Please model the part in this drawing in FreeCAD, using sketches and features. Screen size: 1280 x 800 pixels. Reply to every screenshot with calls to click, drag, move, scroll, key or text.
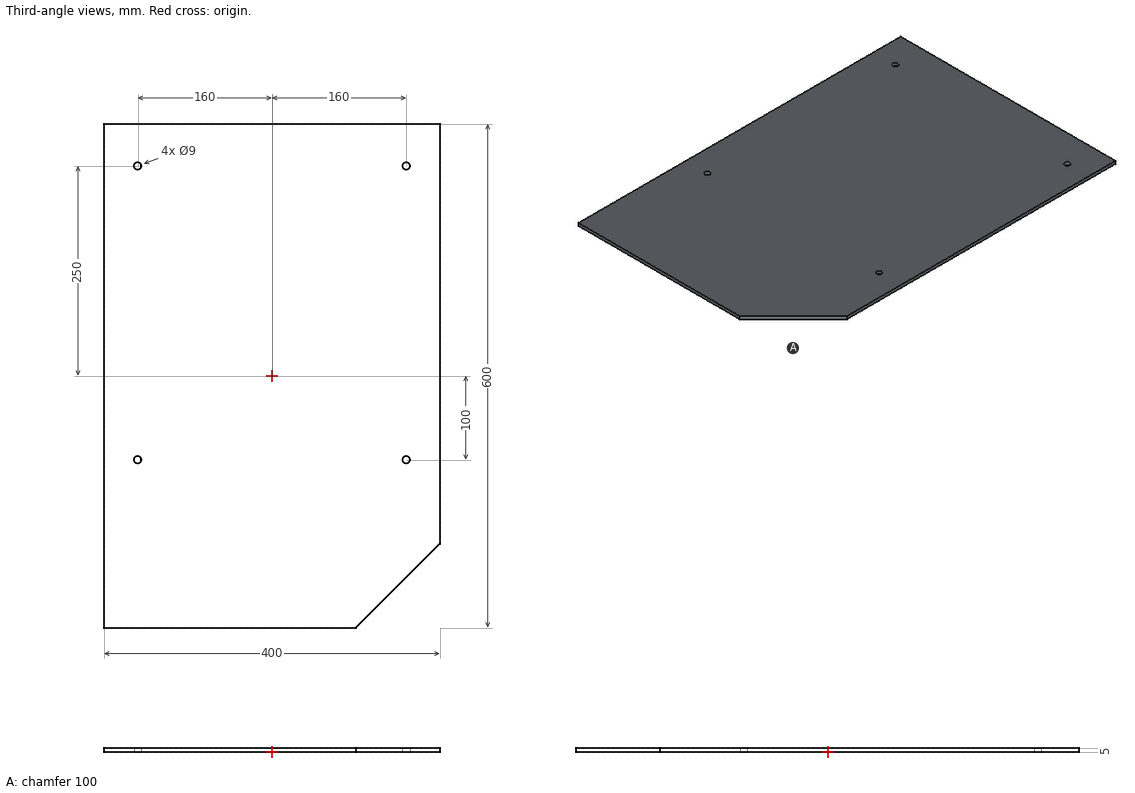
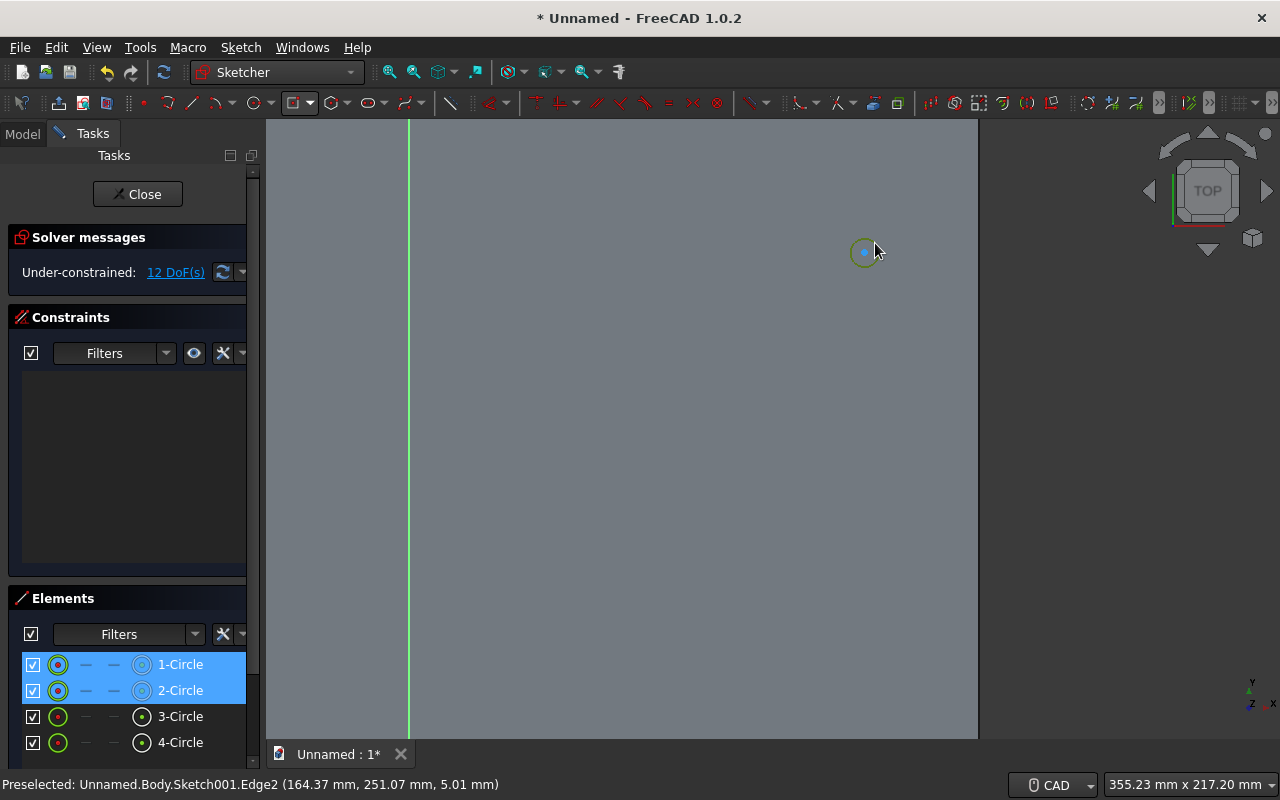
scroll(877, 242, down, 5)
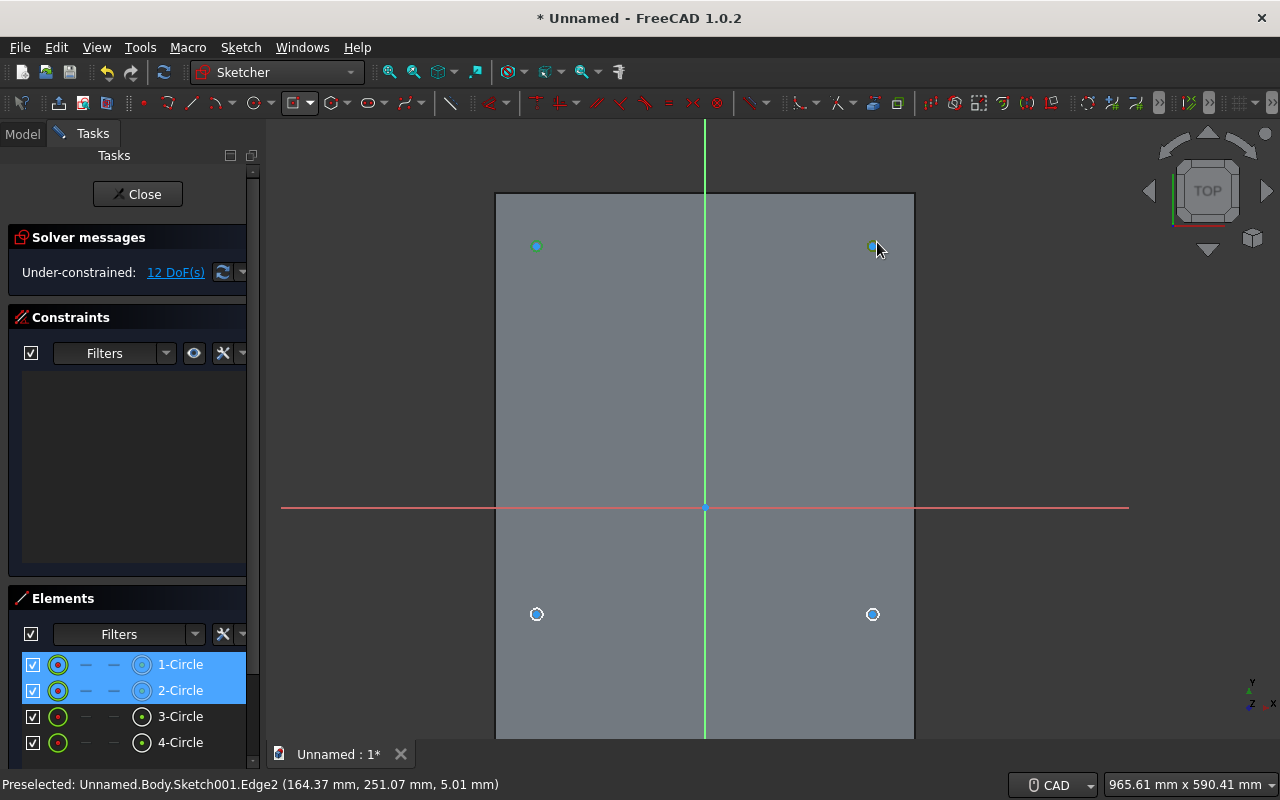
scroll(877, 610, up, 5)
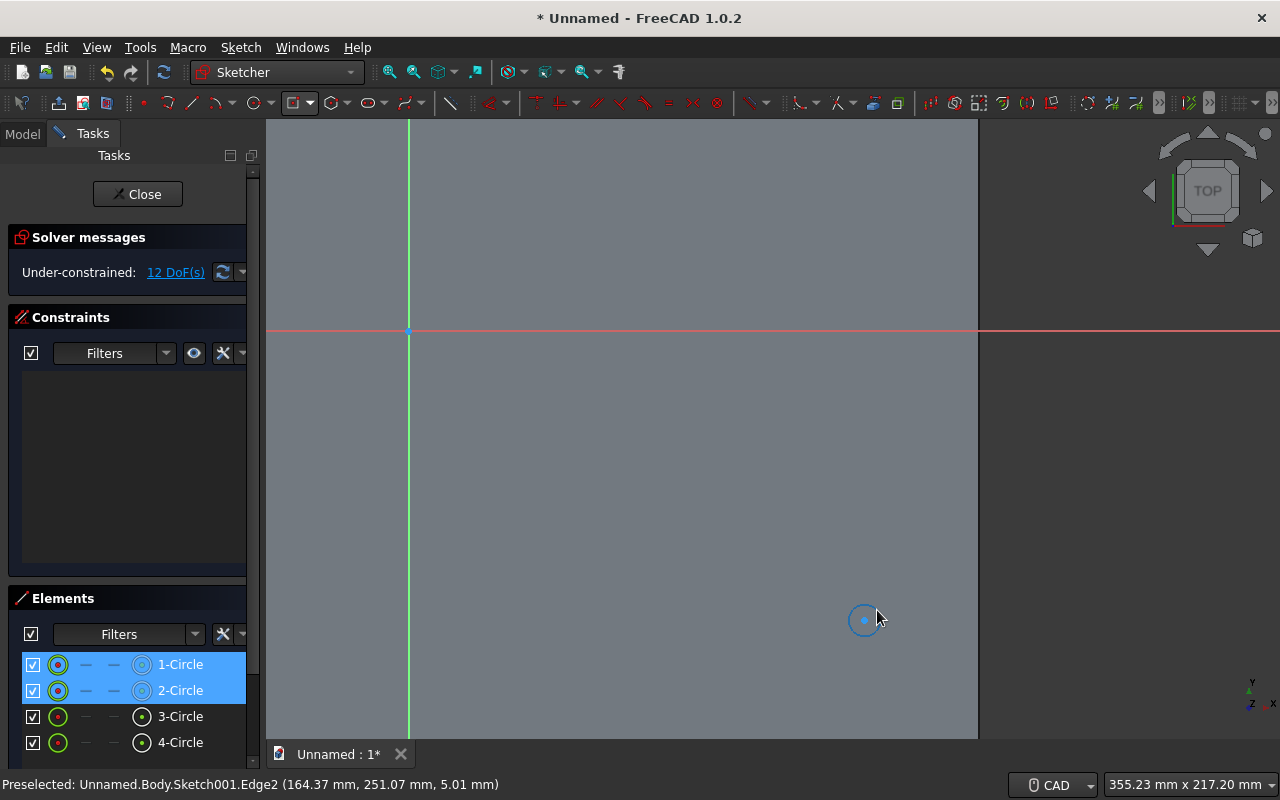
click(876, 609)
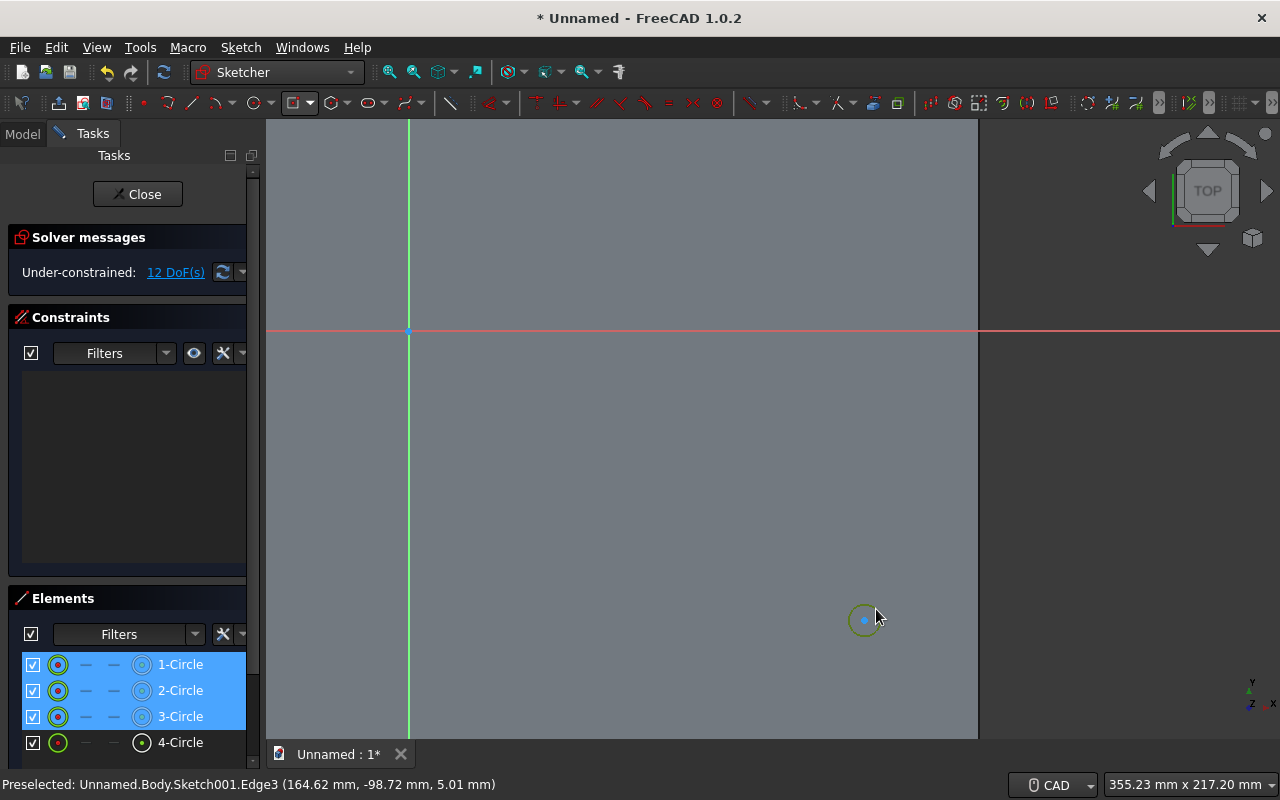
scroll(877, 611, down, 5)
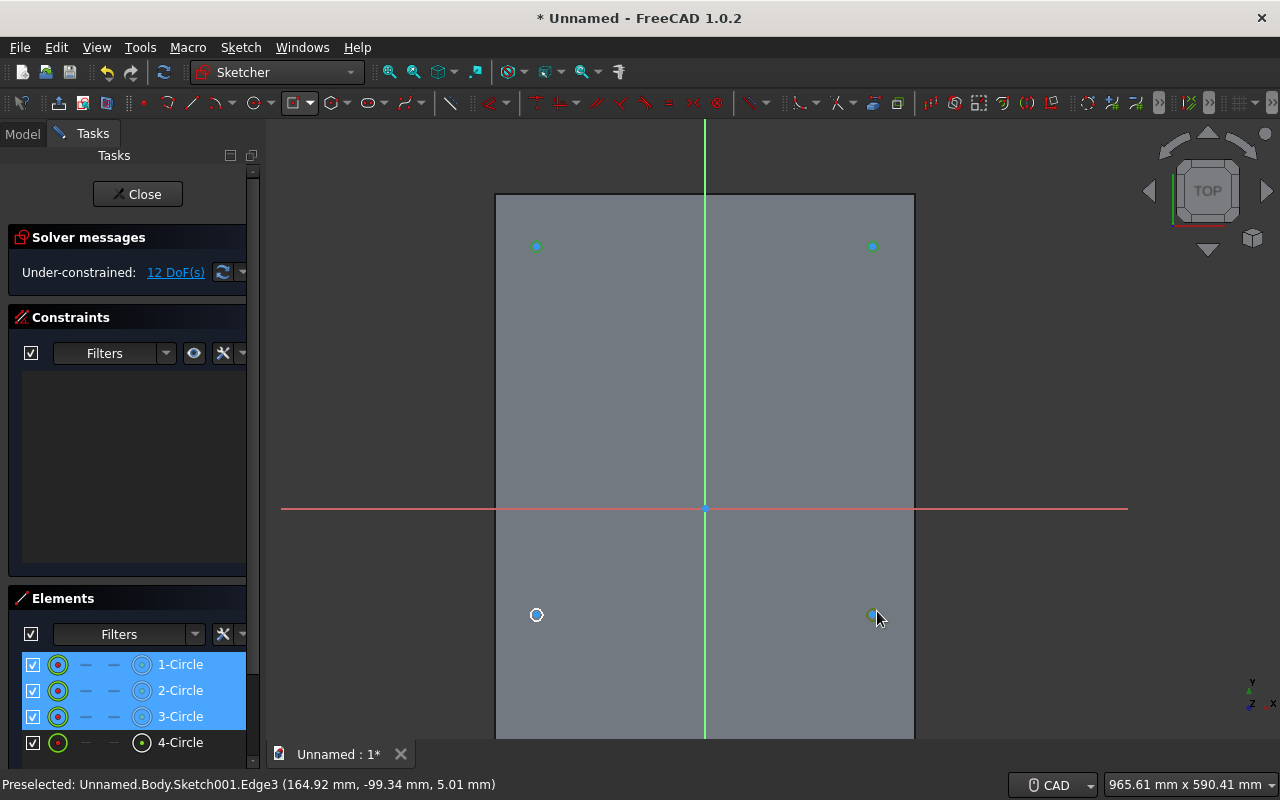
scroll(541, 611, up, 5)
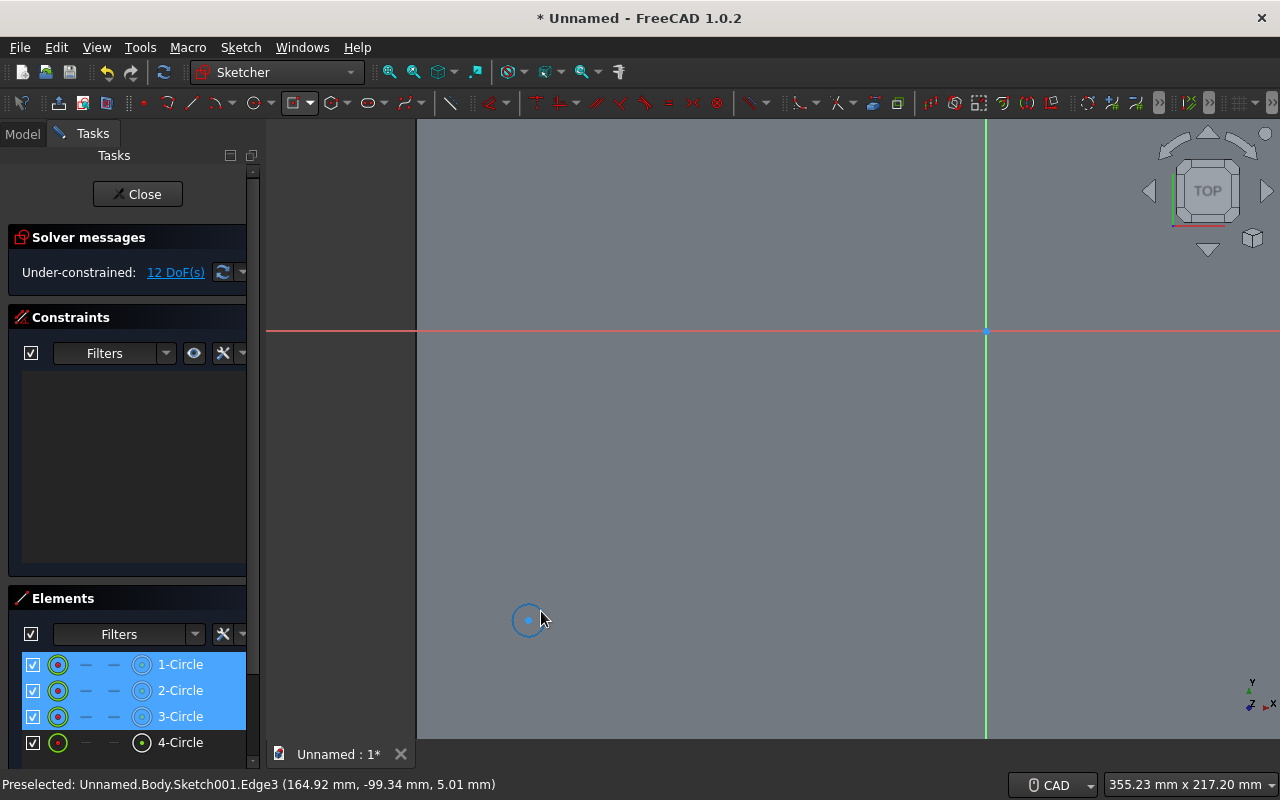
click(540, 609)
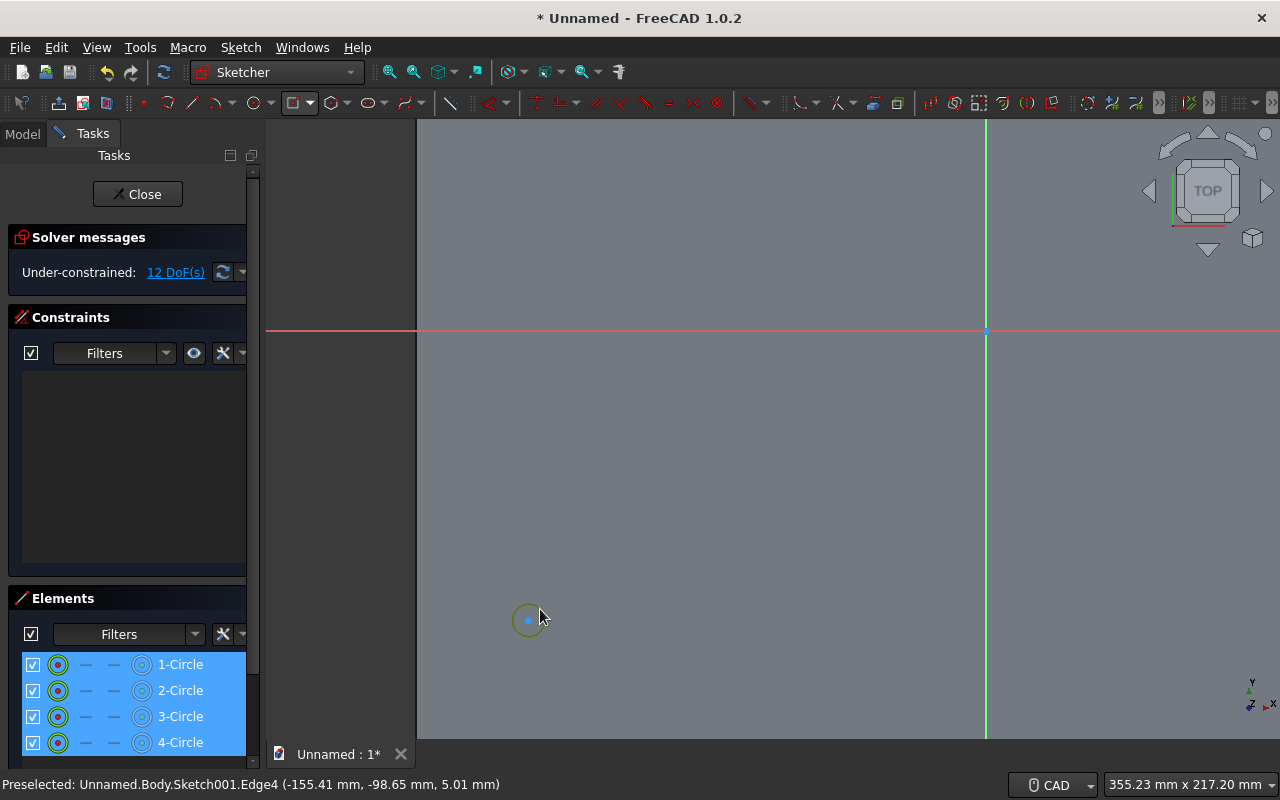
click(670, 104)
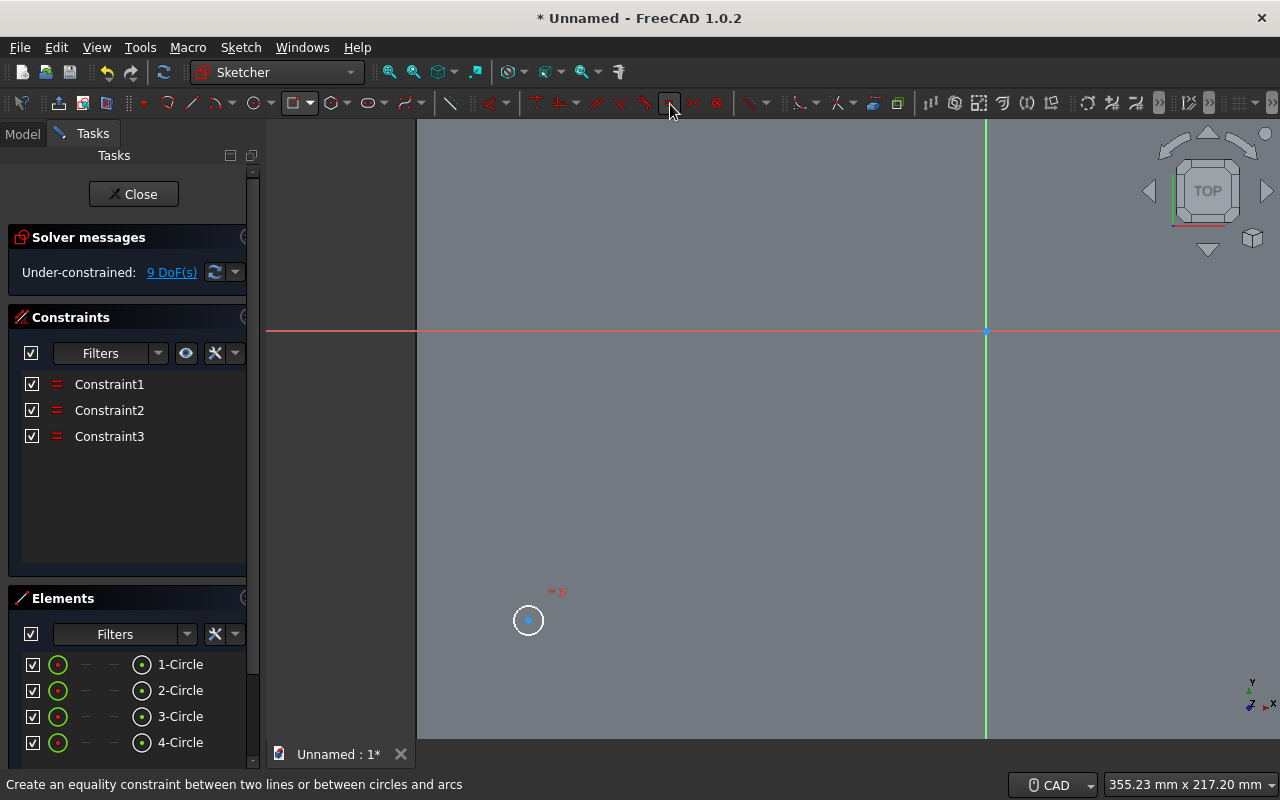
scroll(540, 611, down, 5)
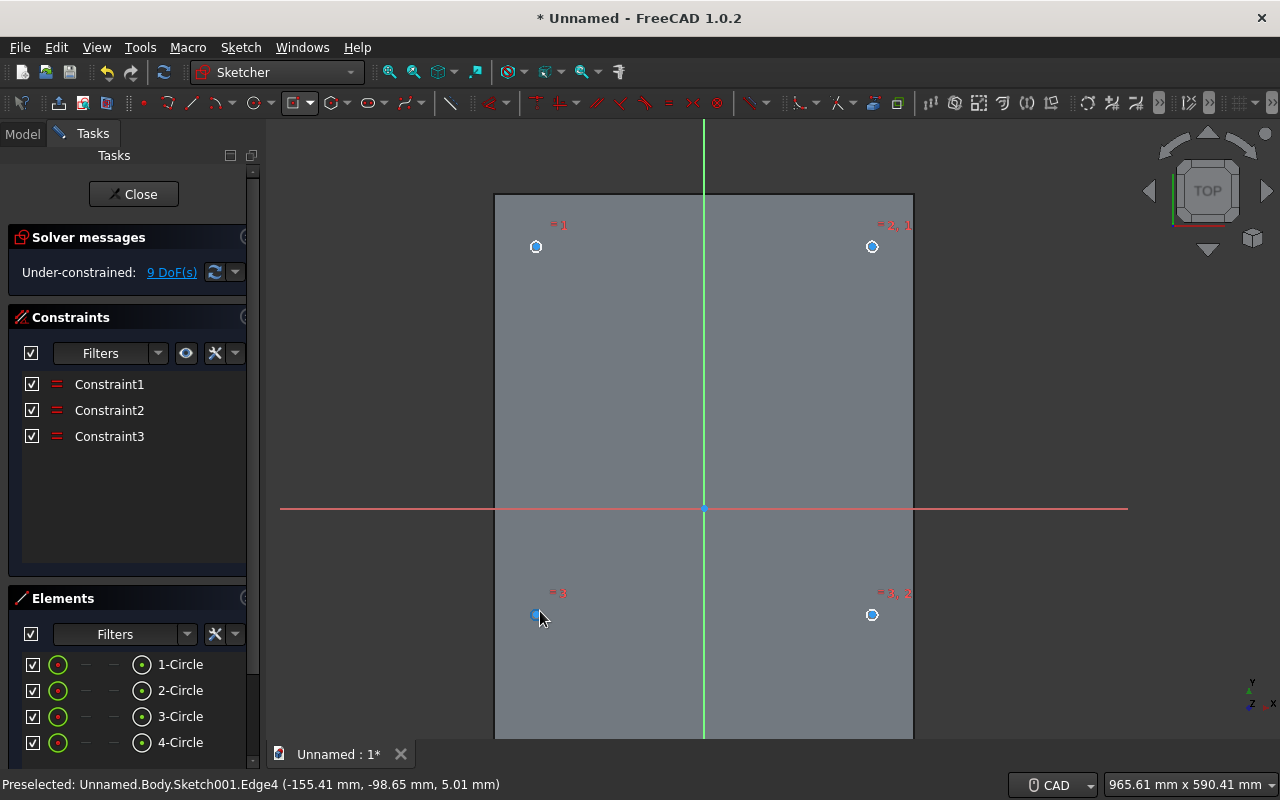
click(536, 247)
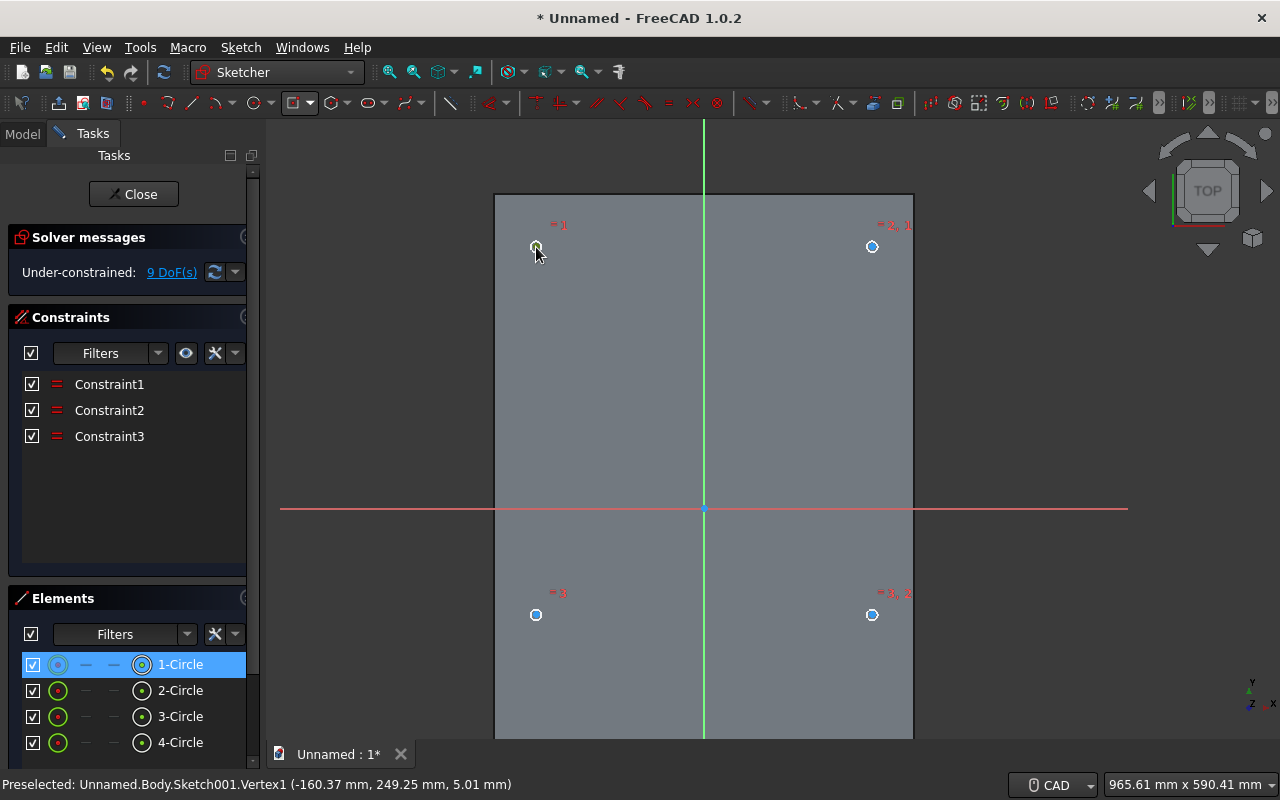
click(872, 247)